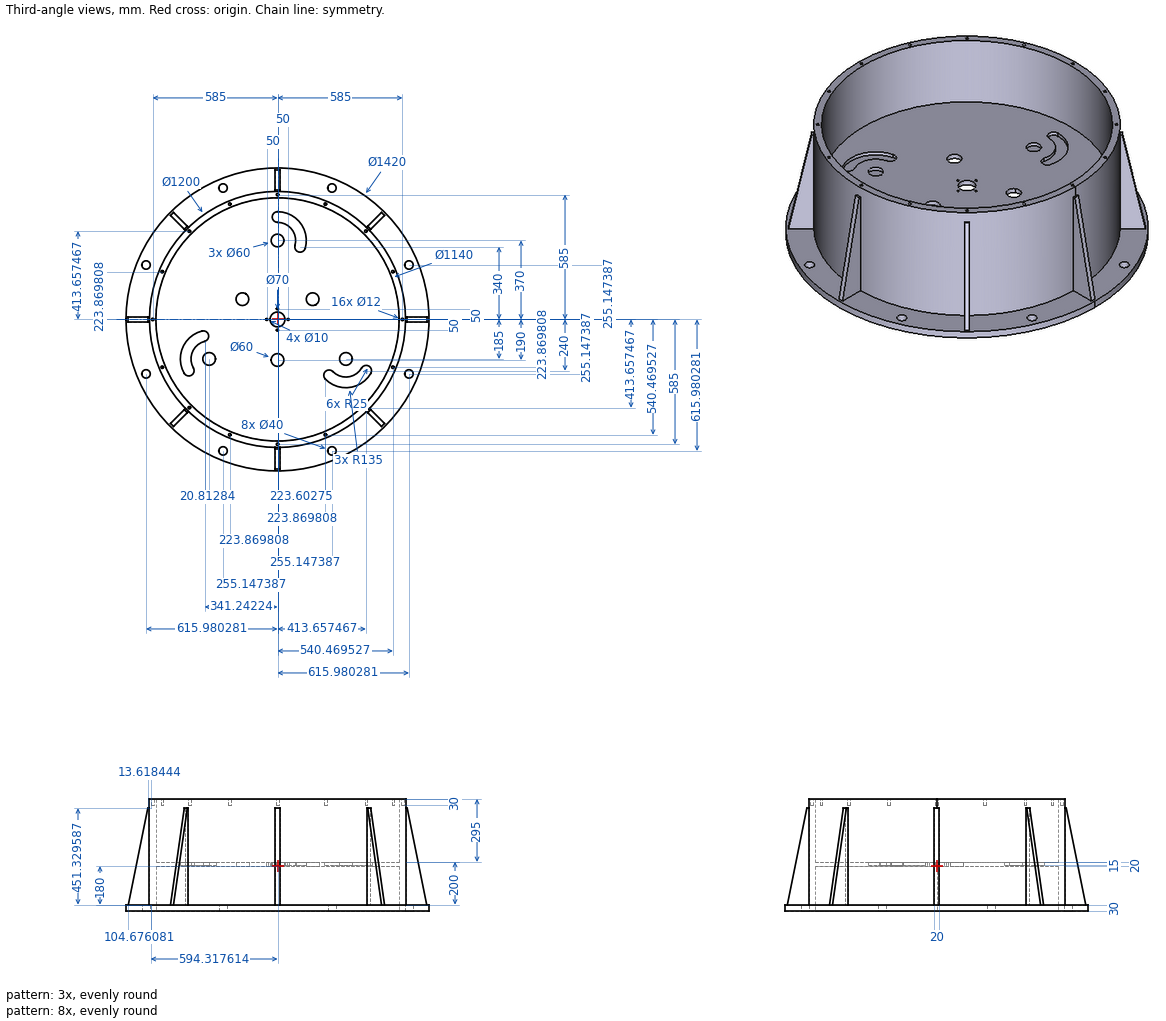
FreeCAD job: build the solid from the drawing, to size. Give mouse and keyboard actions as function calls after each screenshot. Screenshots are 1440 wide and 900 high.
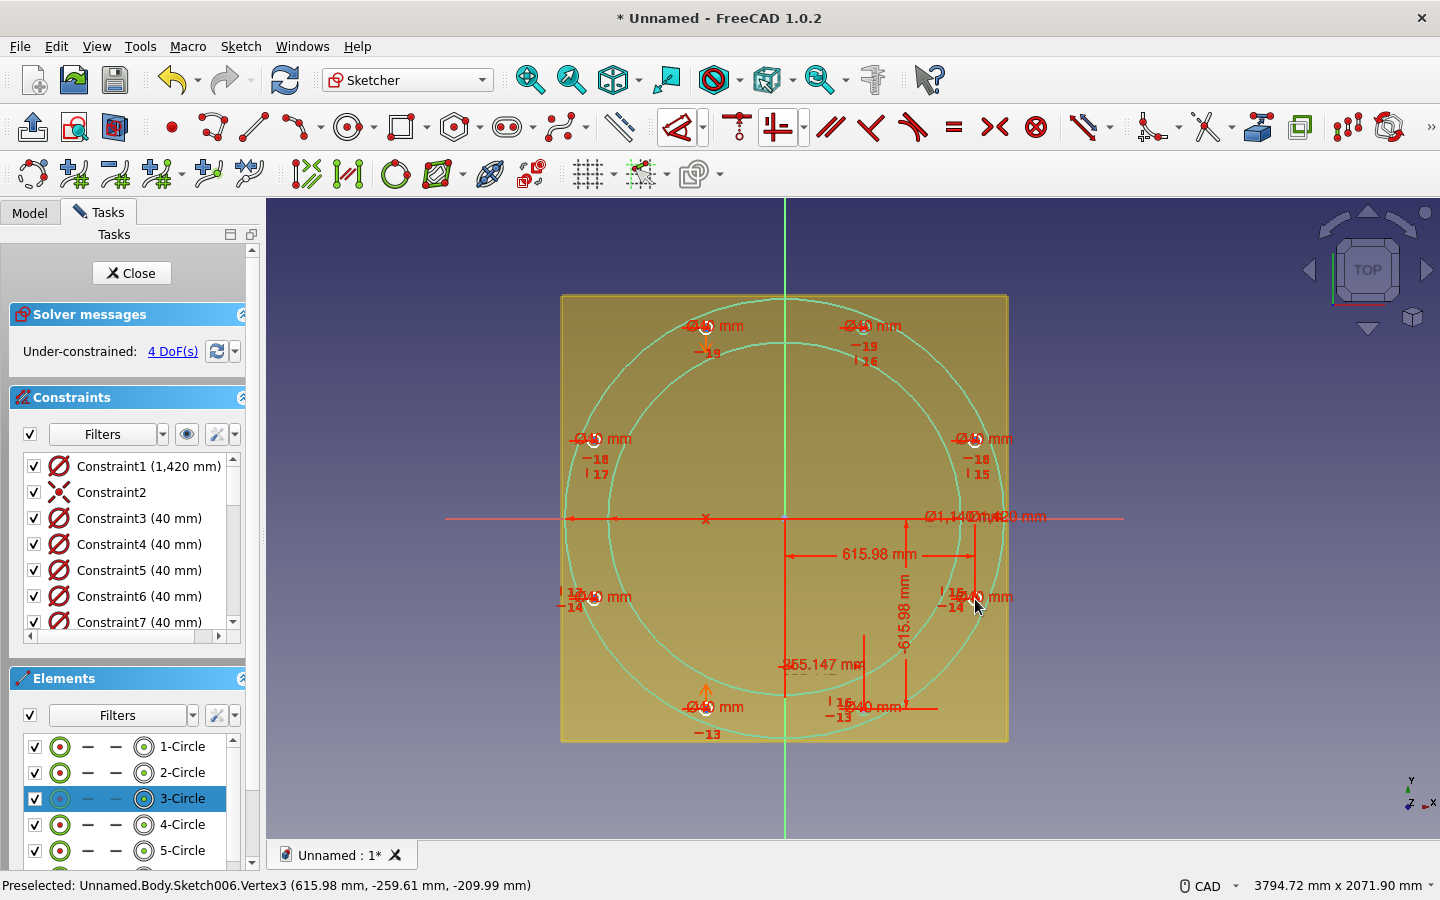
key(i)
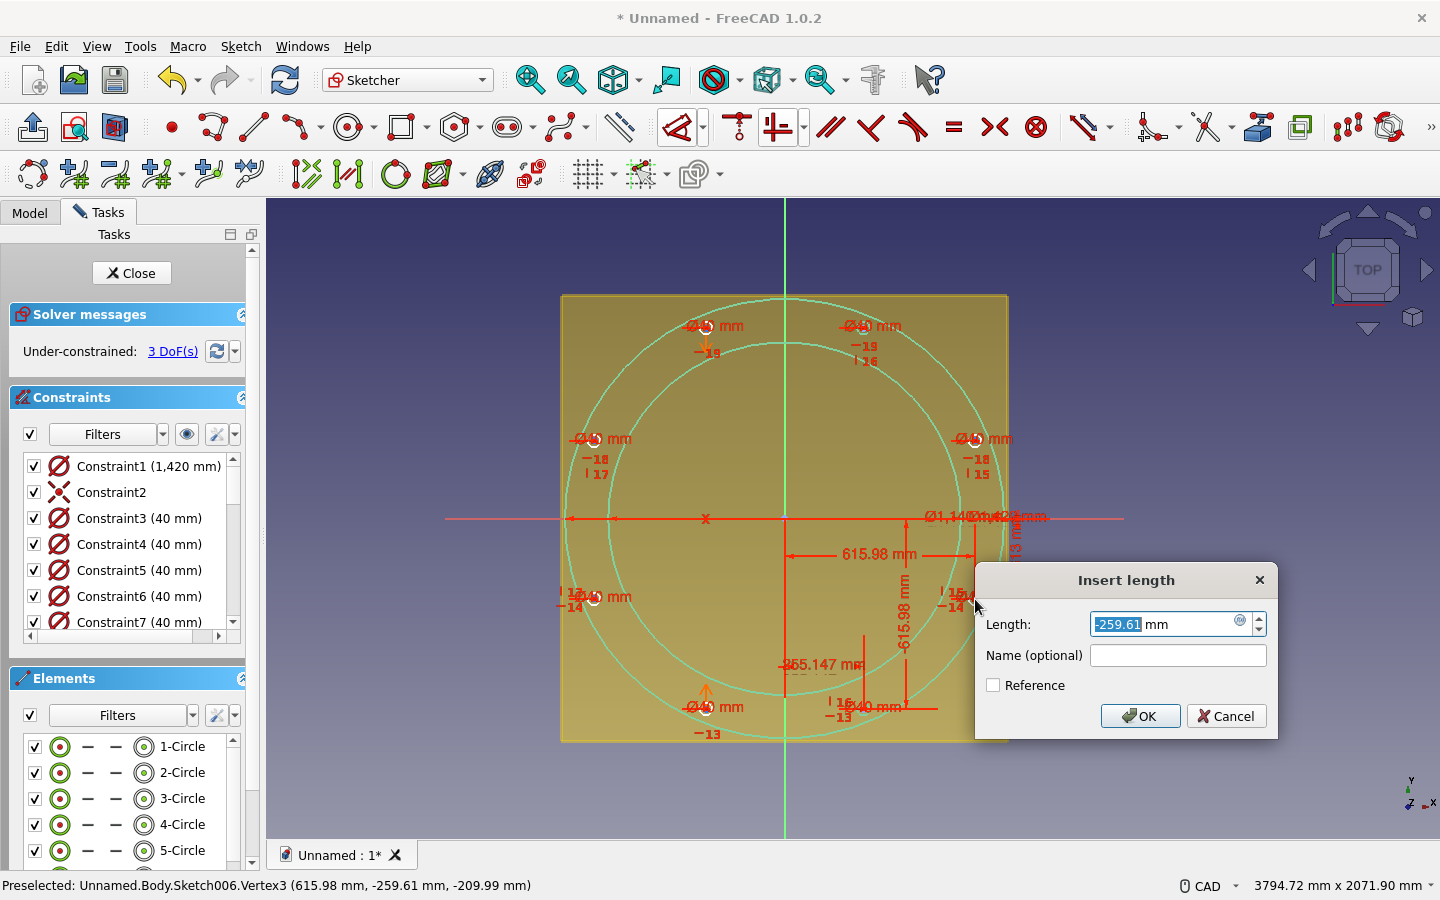
text(-255.147387)
key(Return)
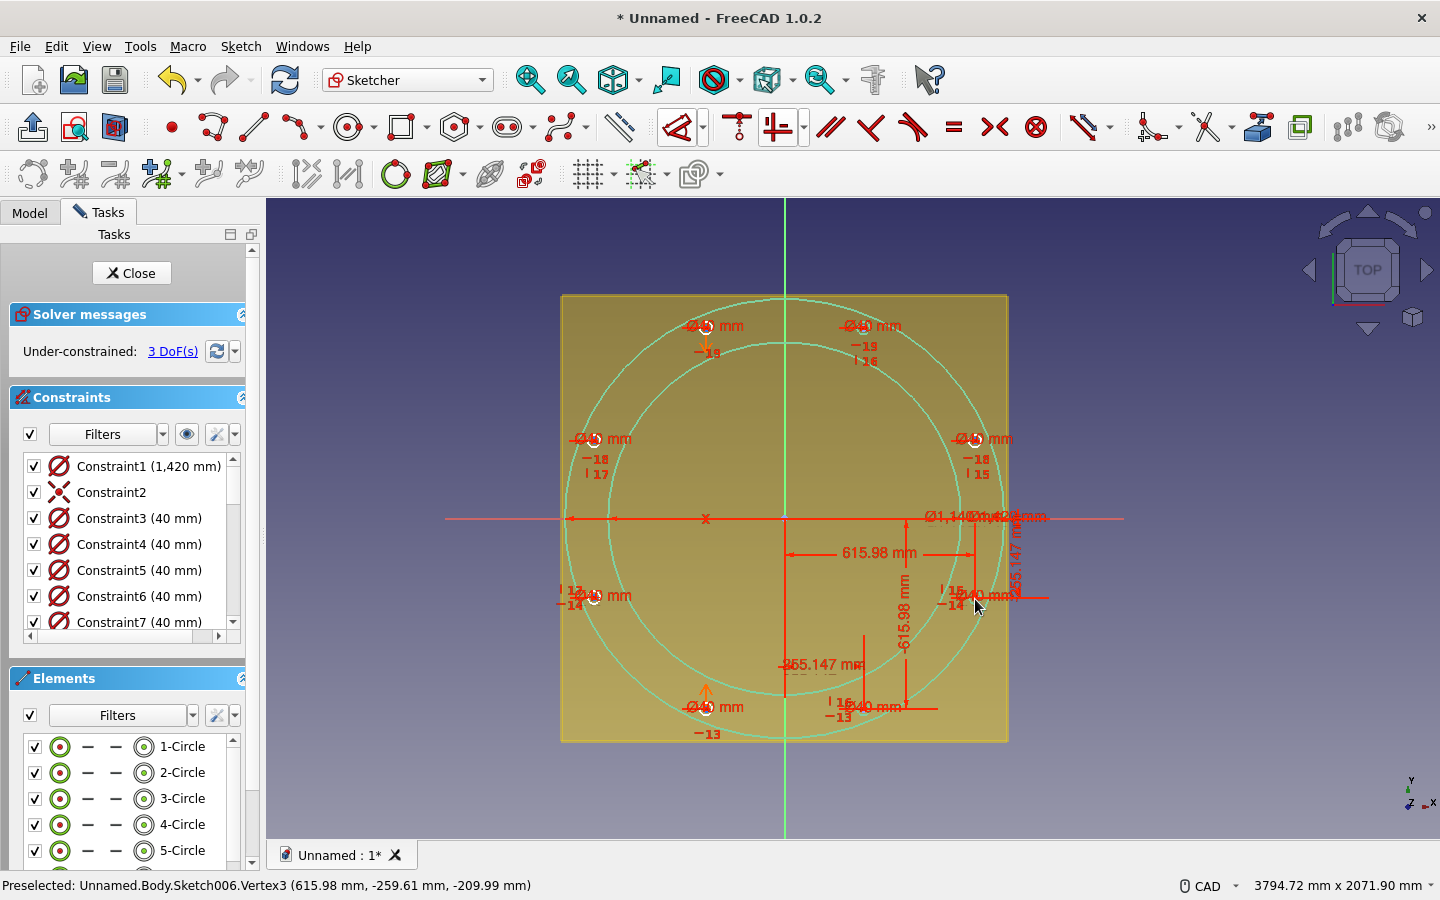
click(706, 709)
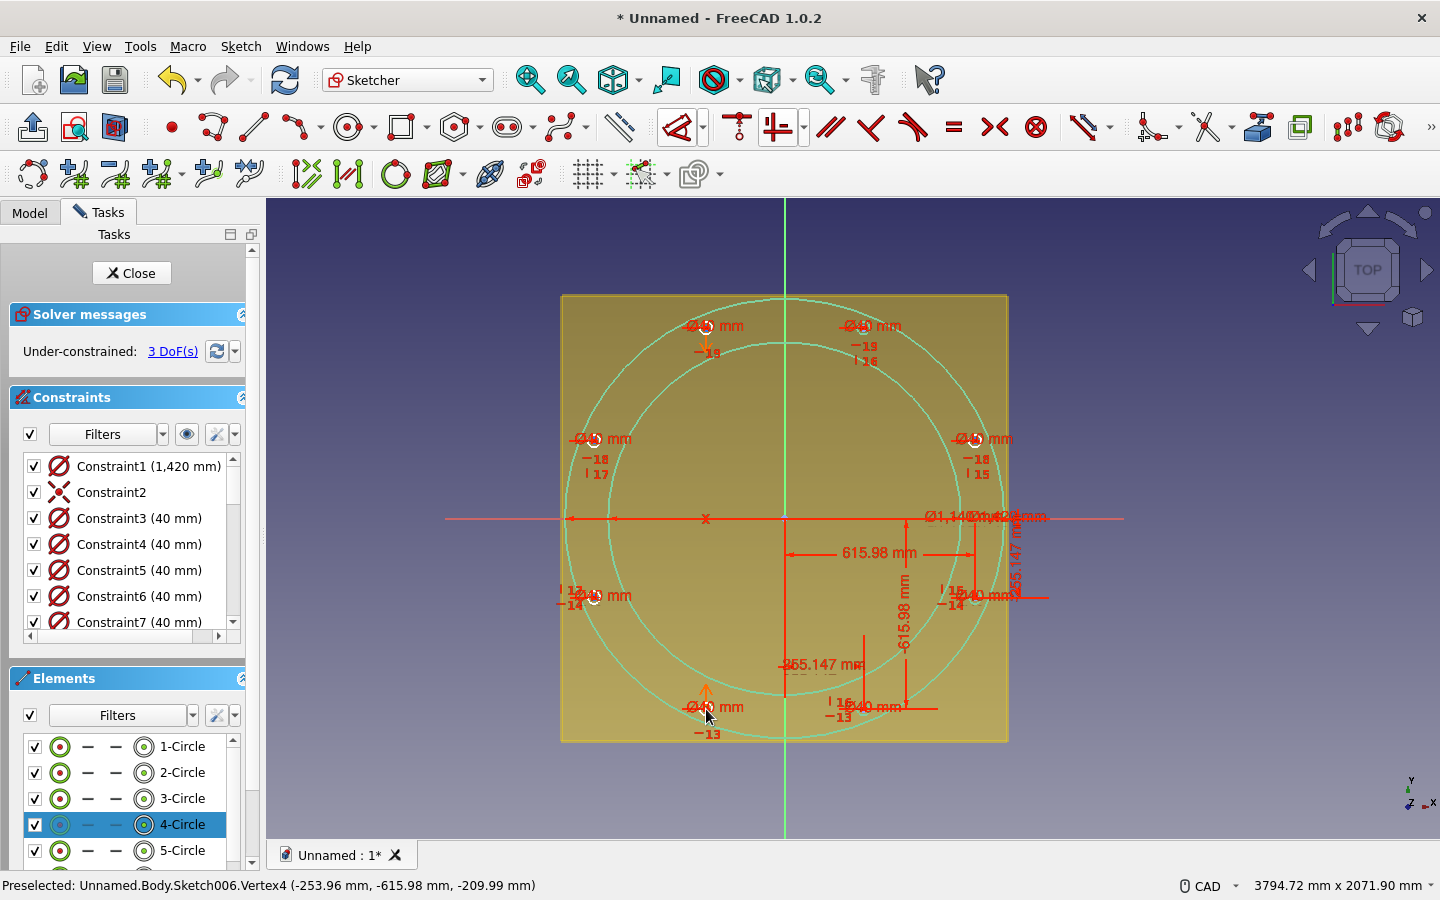
key(l)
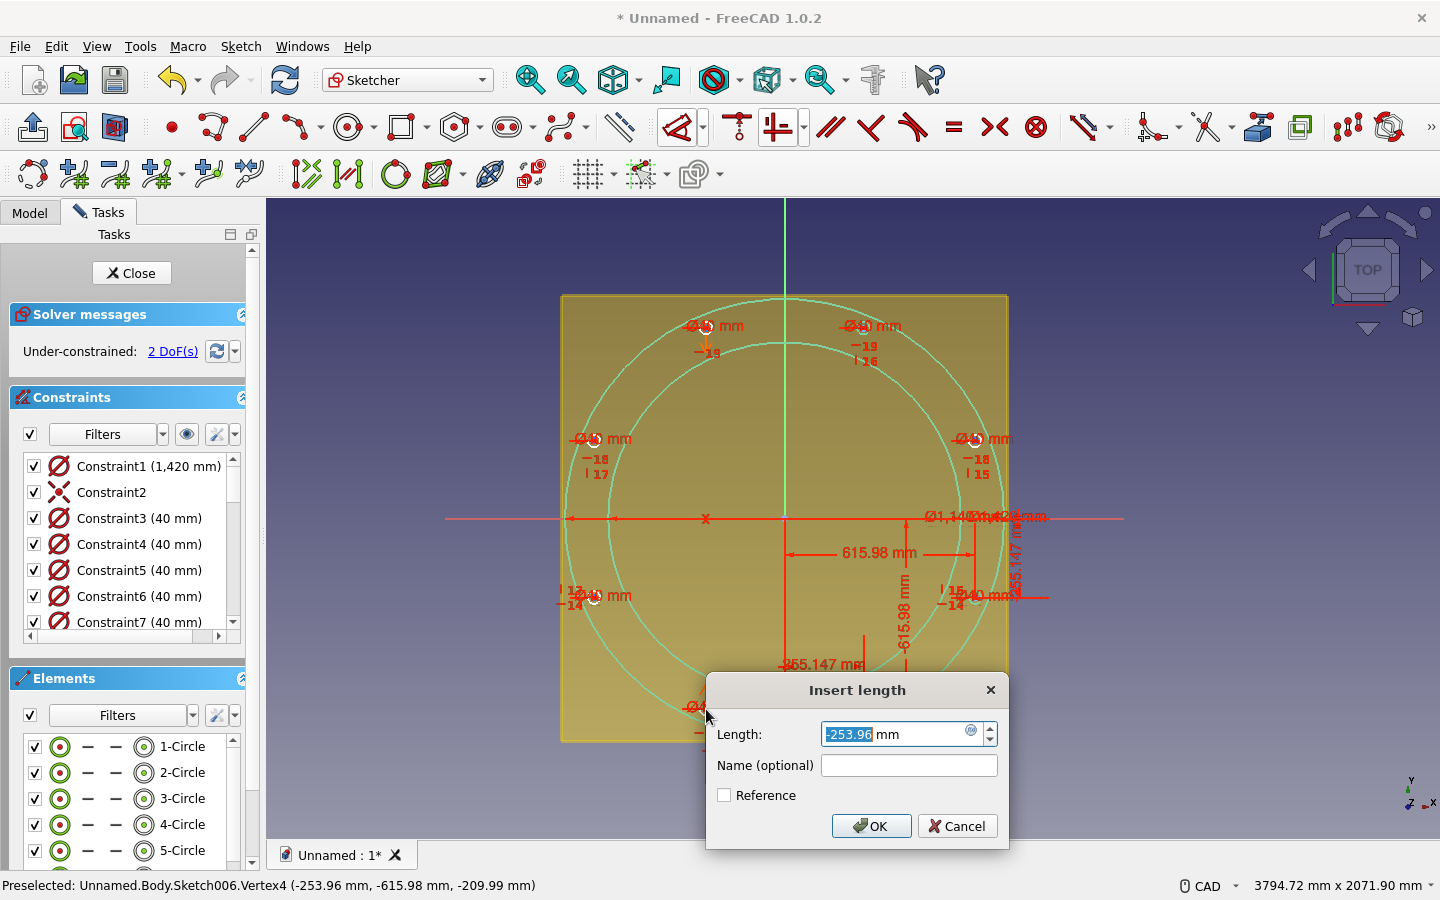
text(-255.147387)
key(Return)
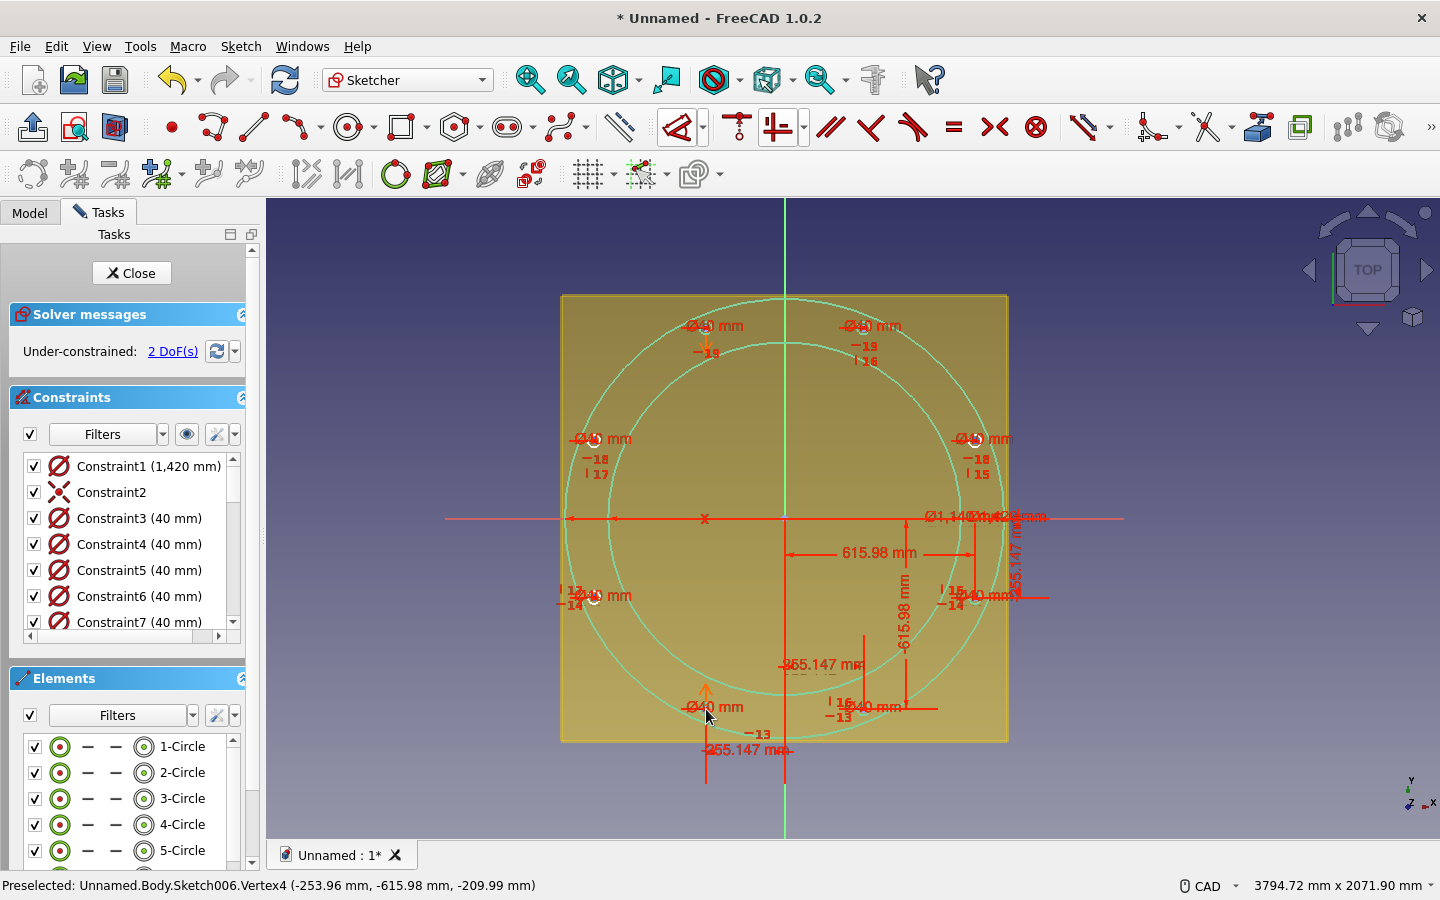
click(594, 598)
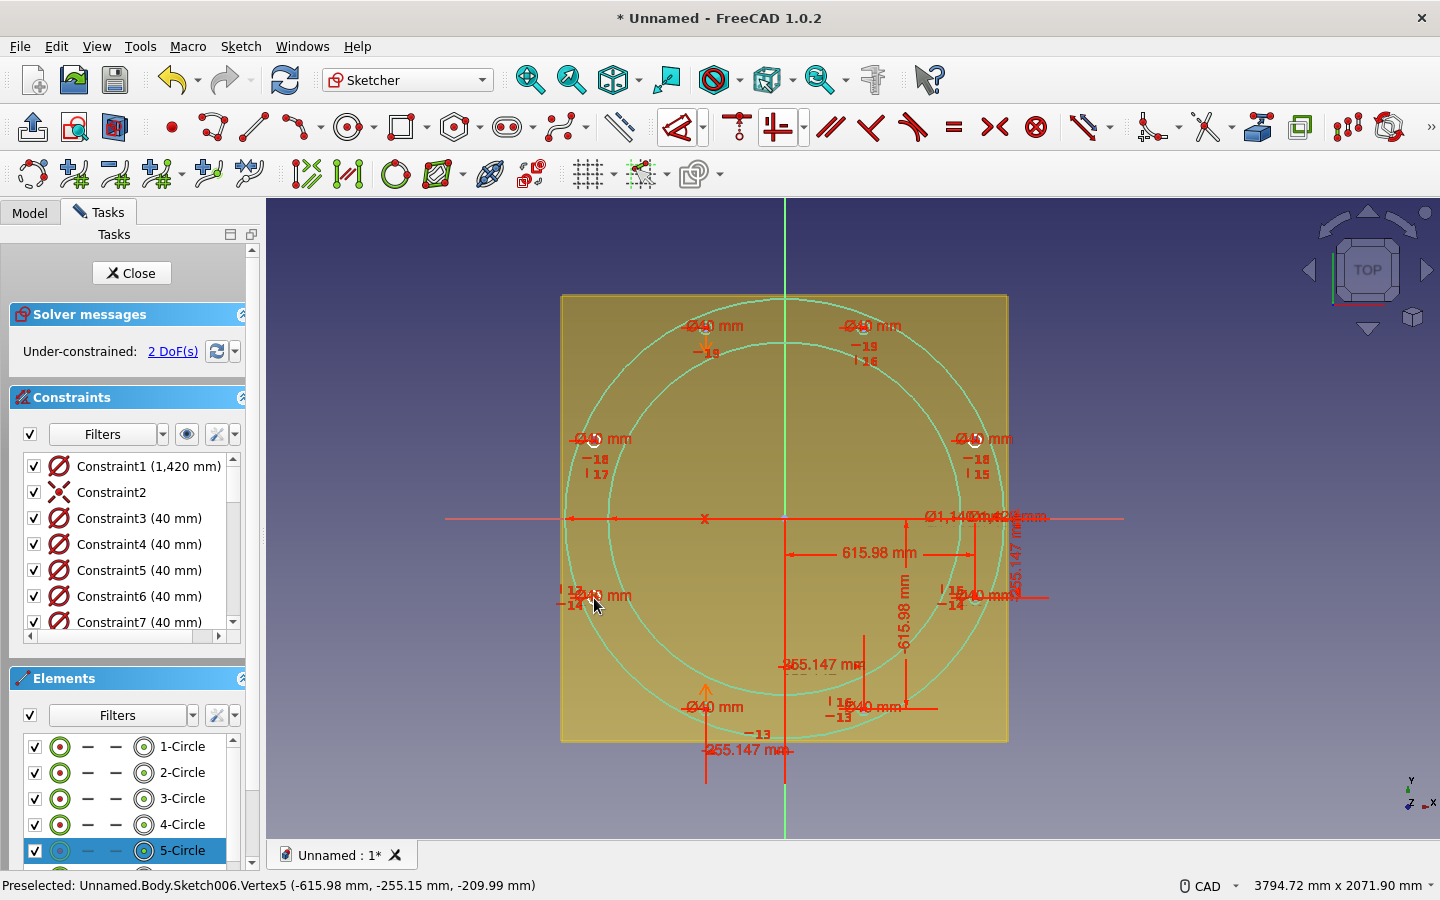
key(l)